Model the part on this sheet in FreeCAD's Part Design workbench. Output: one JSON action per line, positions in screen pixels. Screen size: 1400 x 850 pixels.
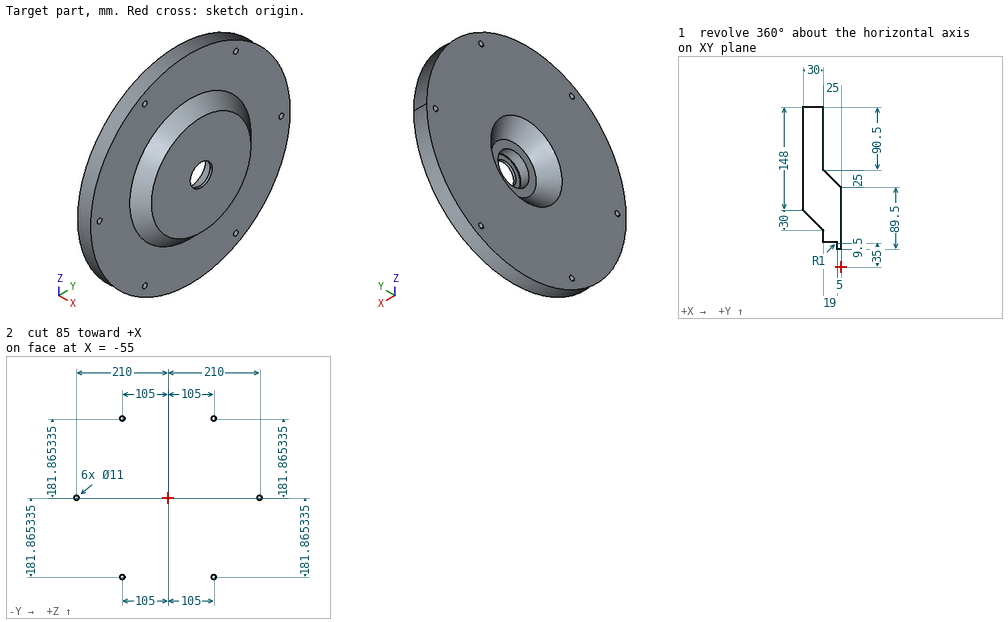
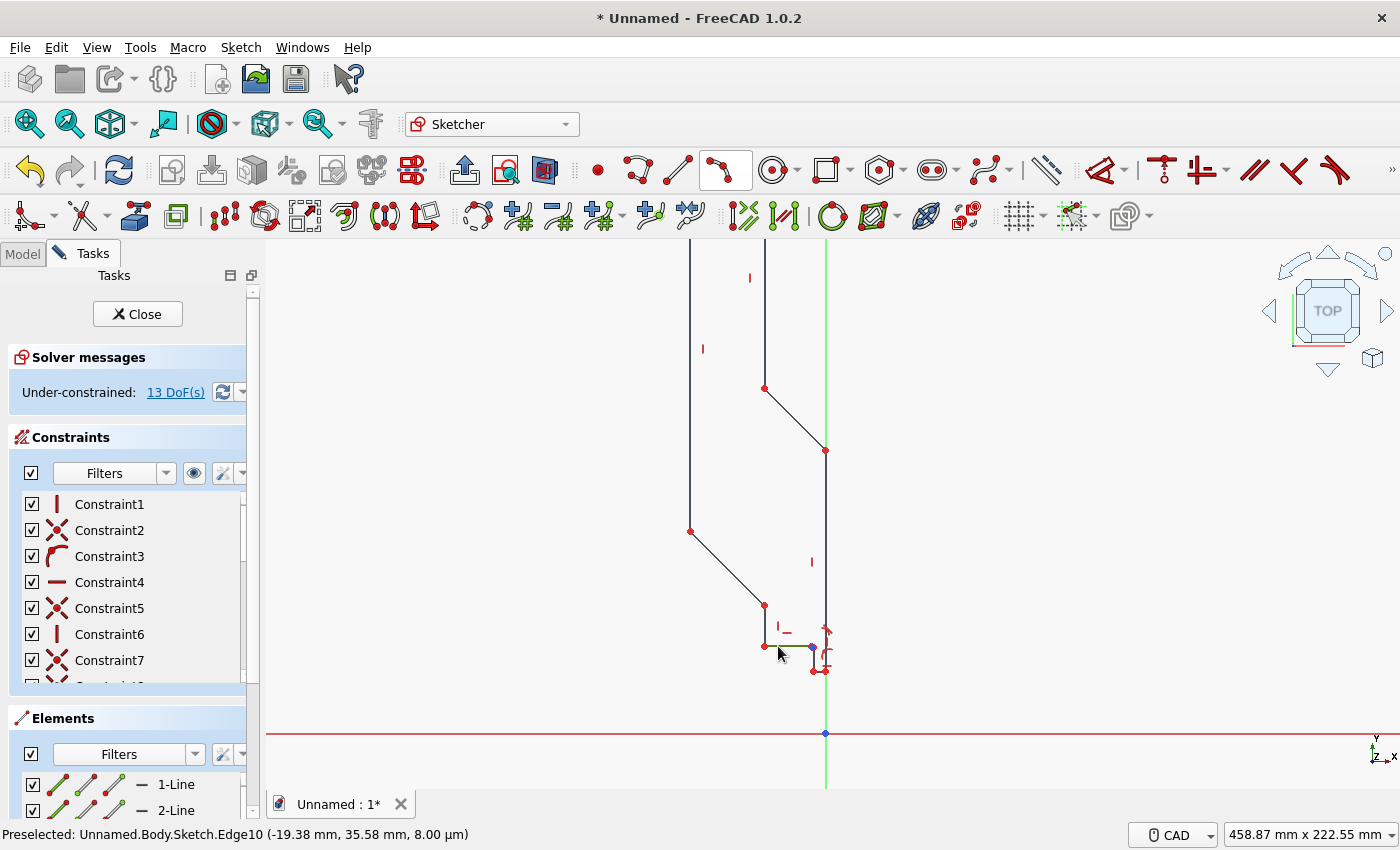
{"action": "scroll", "coordinate": [813, 646], "scroll_direction": "up", "scroll_amount": 11}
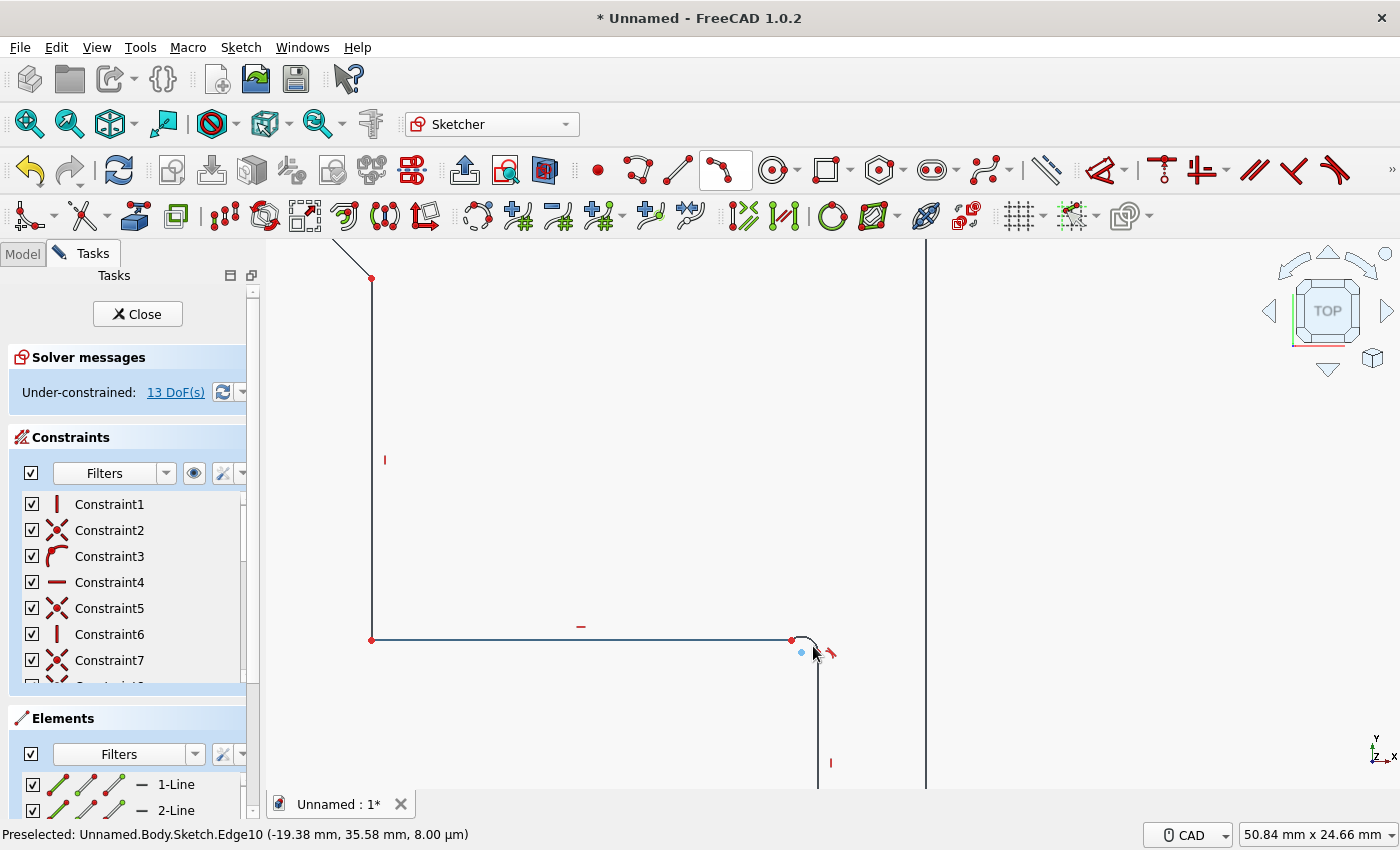
{"action": "left_click", "coordinate": [808, 638]}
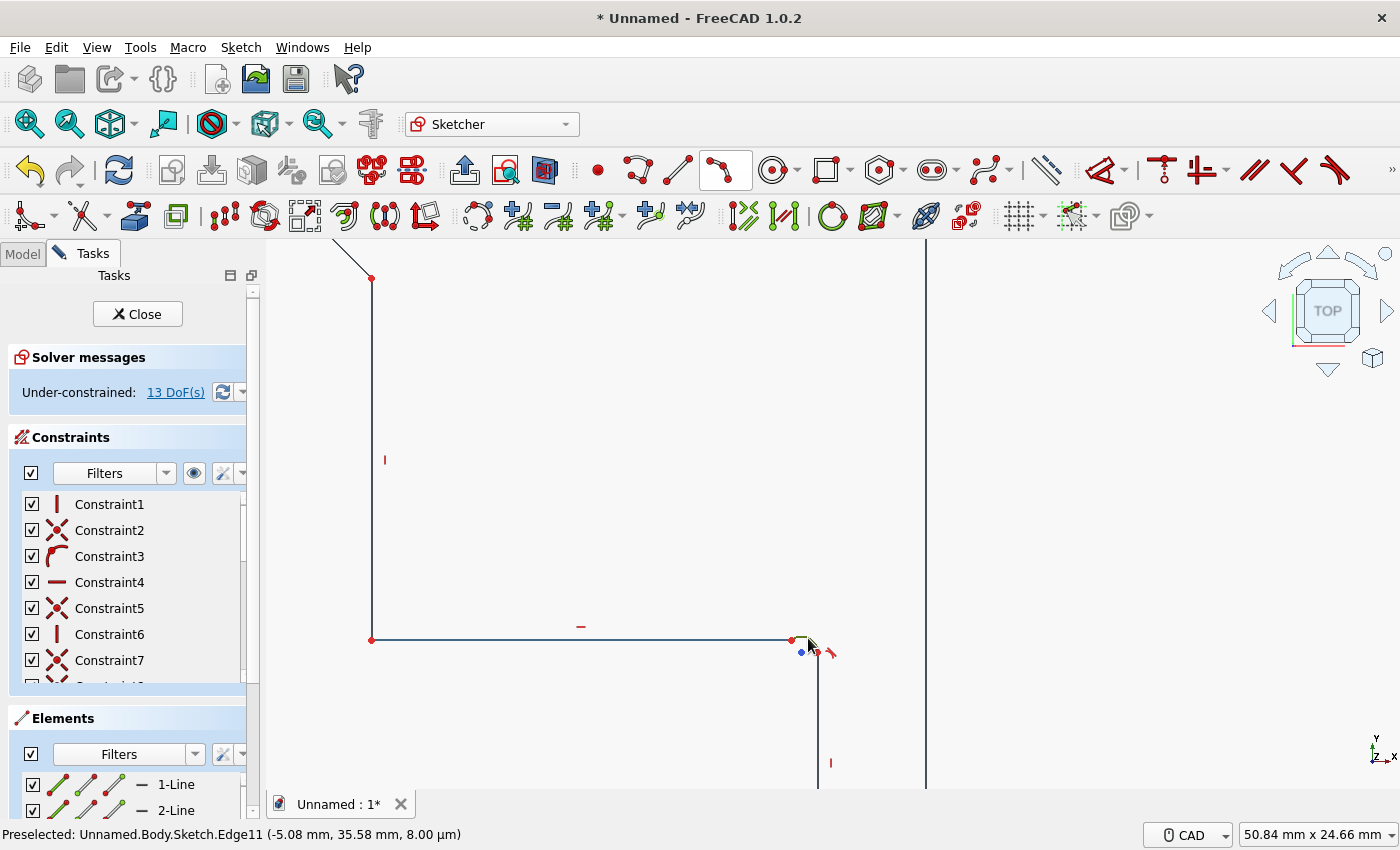
{"action": "left_click", "coordinate": [1336, 170]}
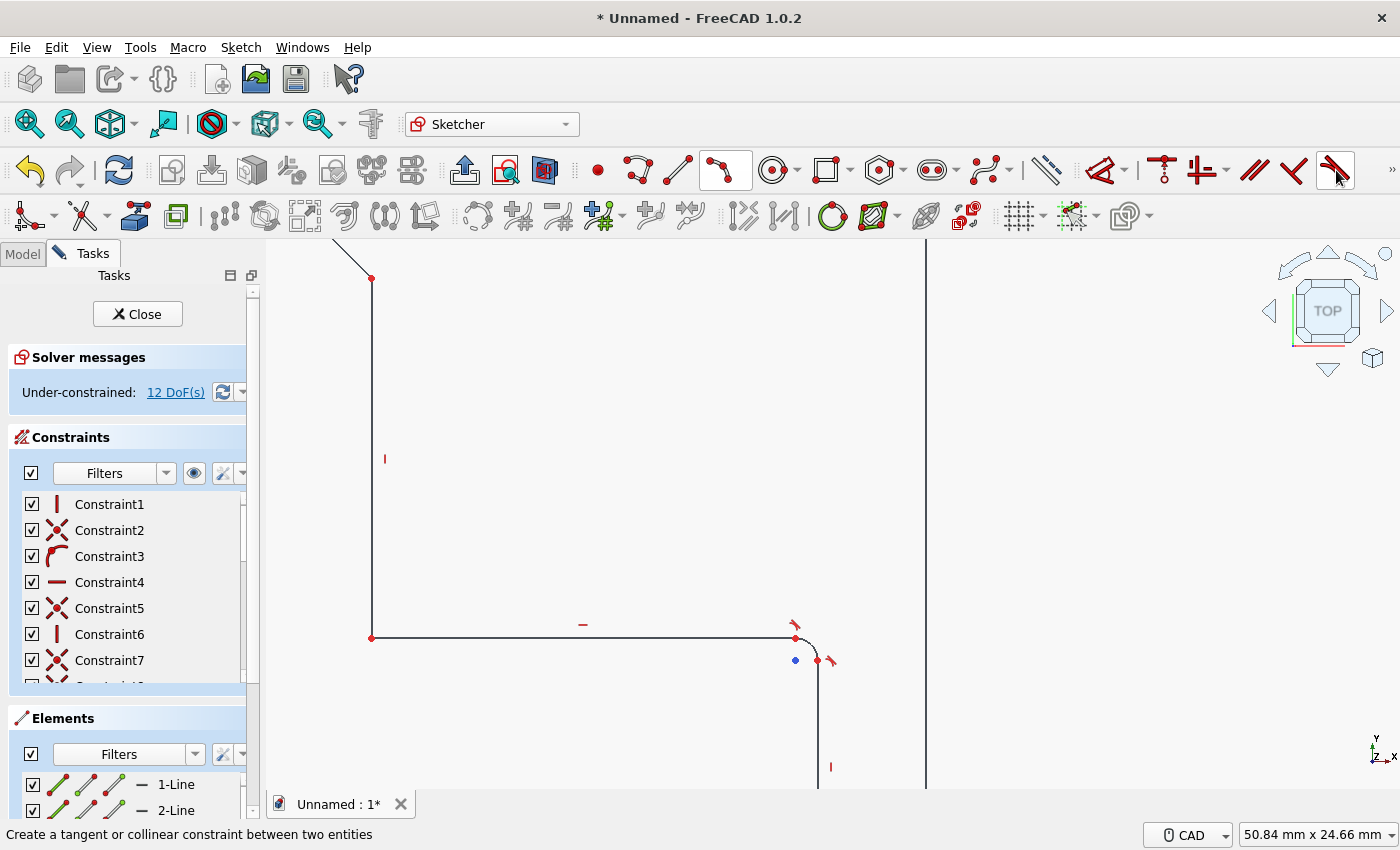
{"action": "left_click", "coordinate": [1100, 170]}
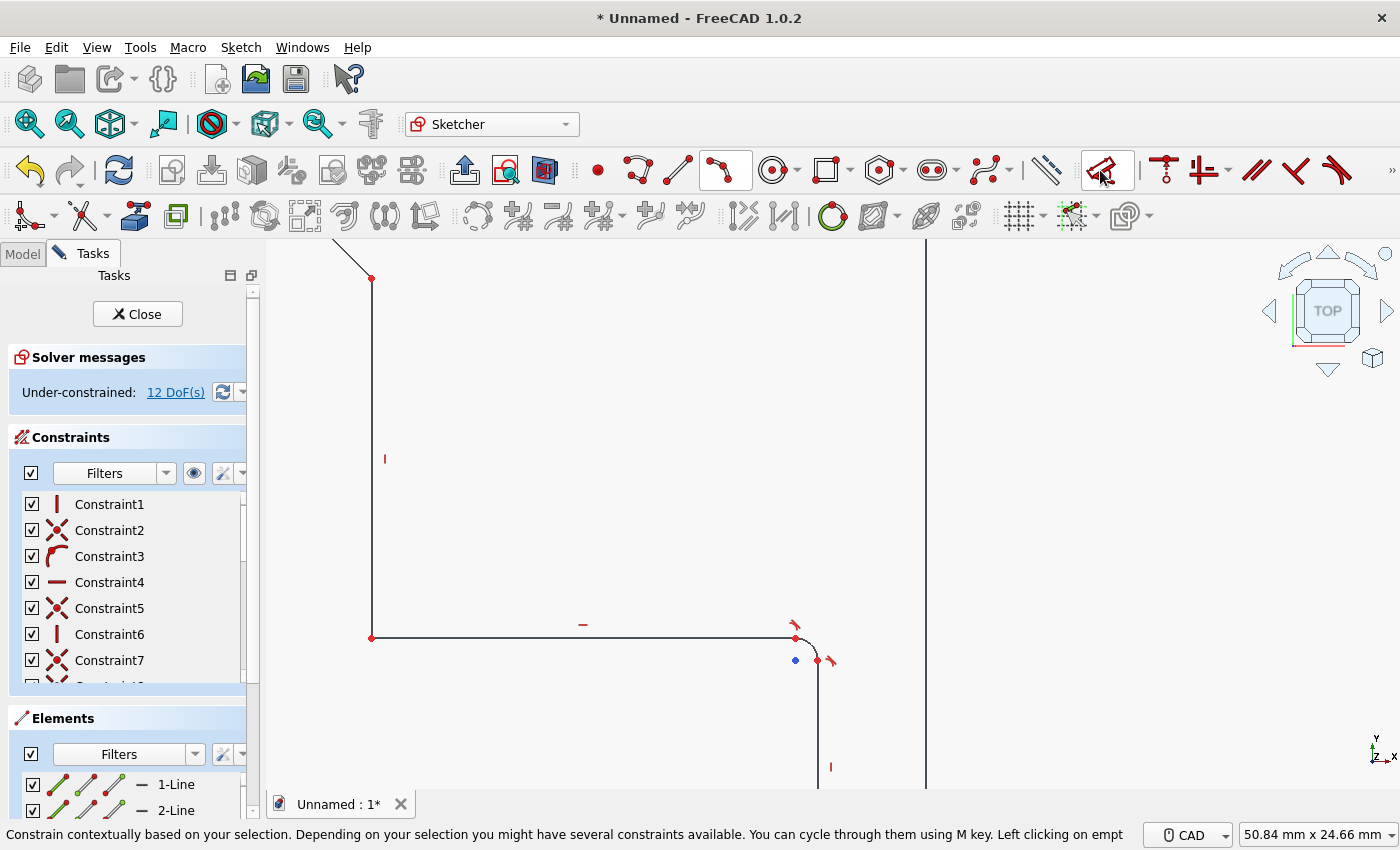
{"action": "scroll", "coordinate": [815, 651], "scroll_direction": "up", "scroll_amount": 3}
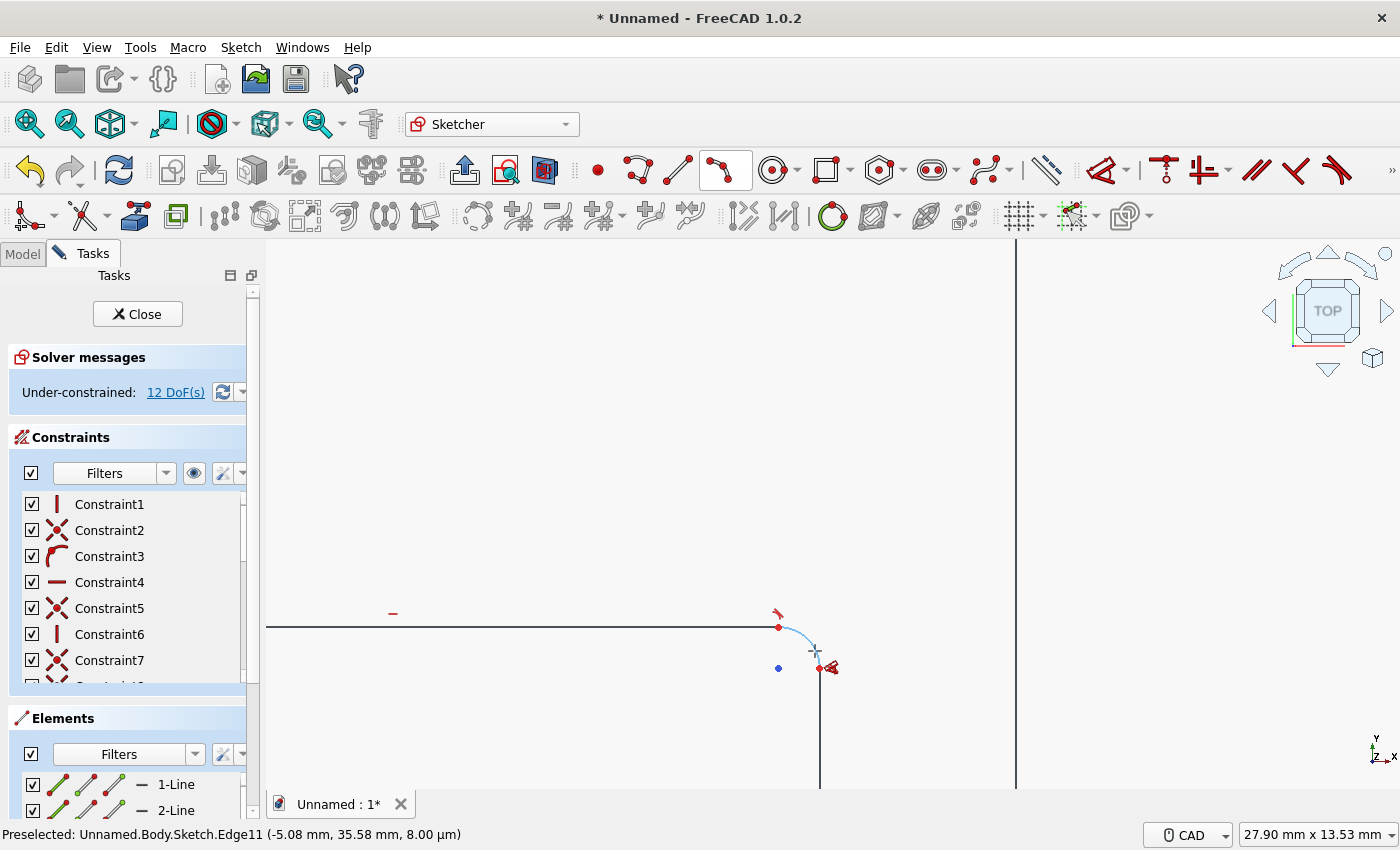
{"action": "left_click", "coordinate": [815, 650]}
{"action": "left_click", "coordinate": [844, 636]}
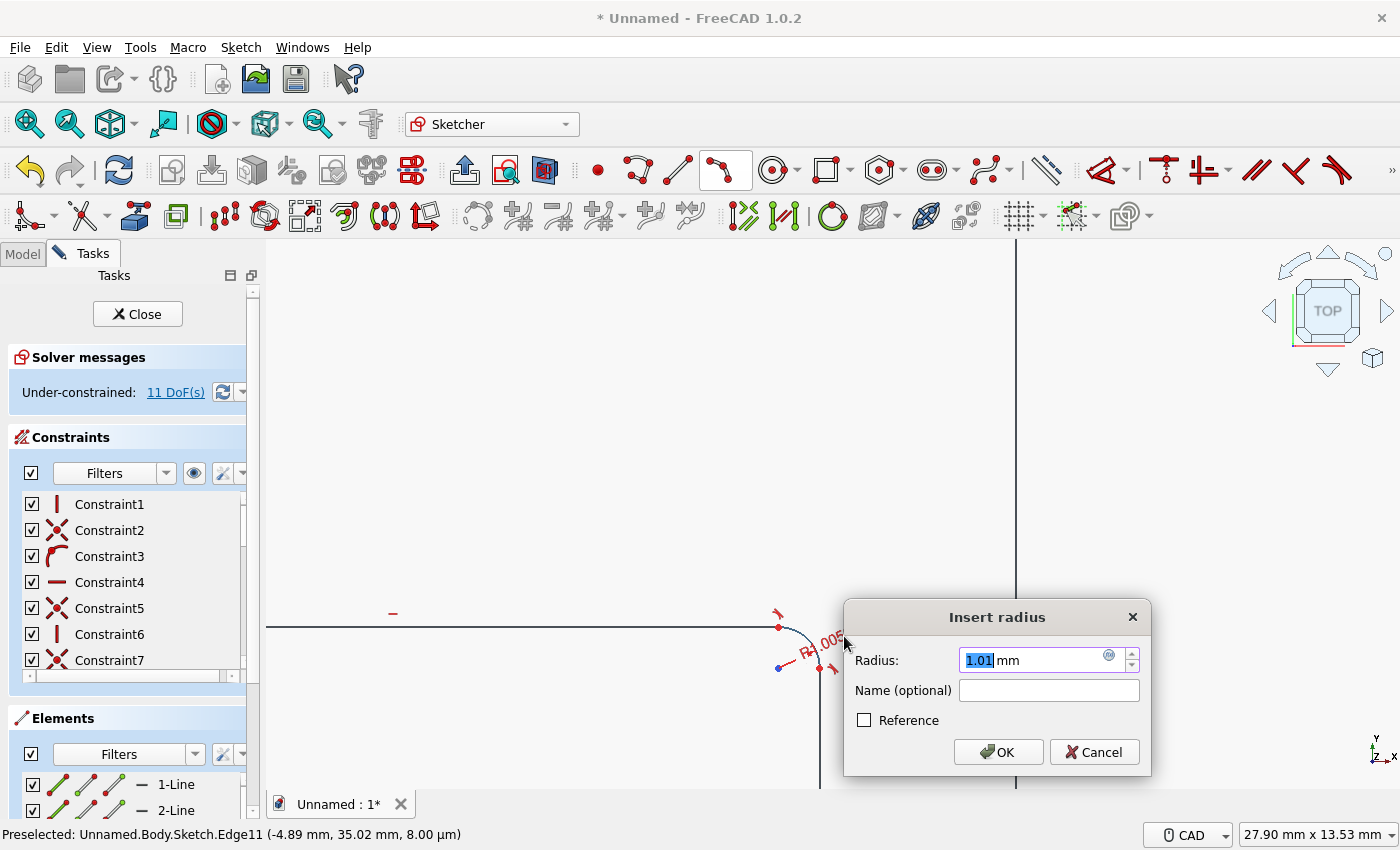
{"action": "type", "text": "1"}
{"action": "key", "text": "Return"}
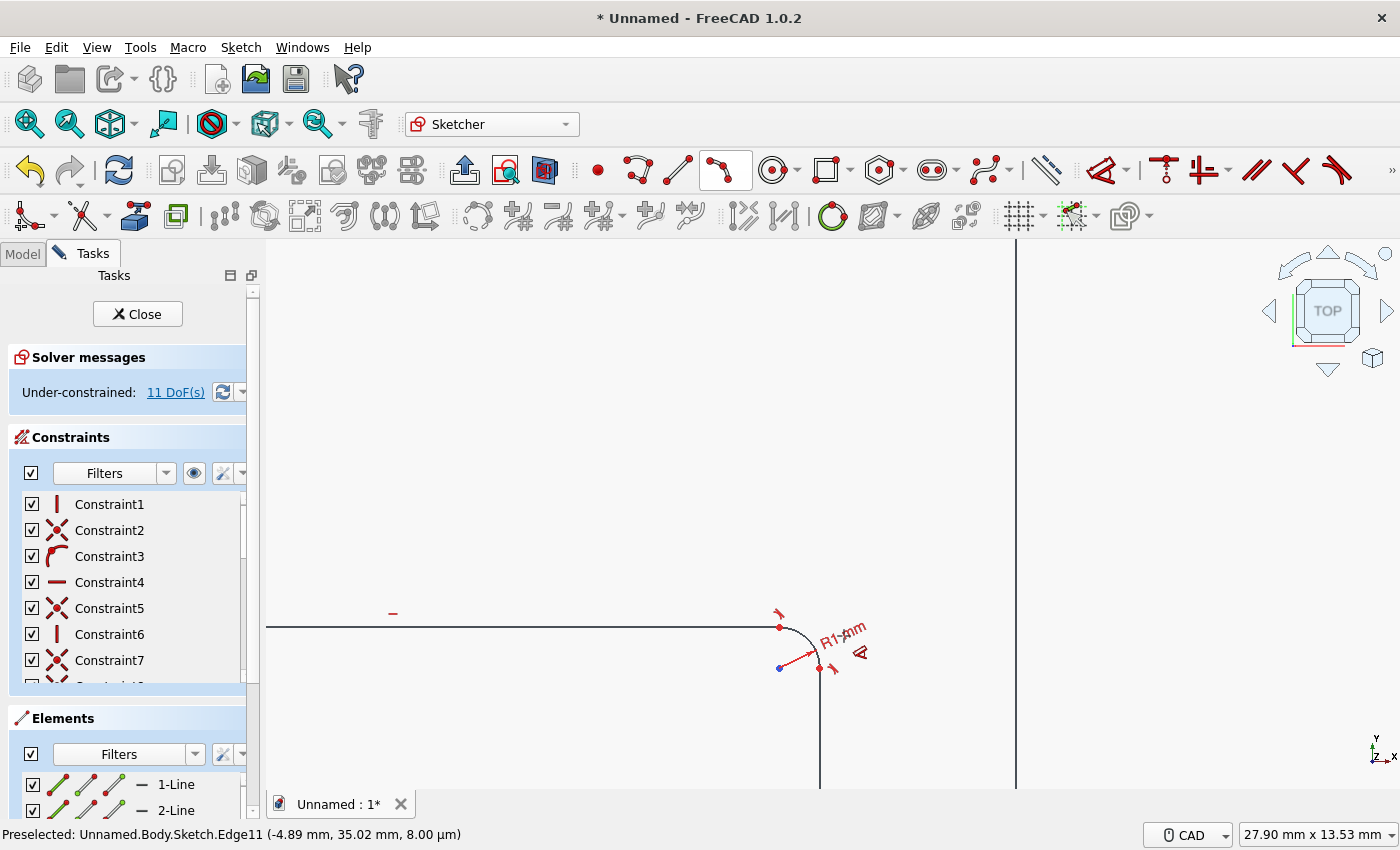
{"action": "scroll", "coordinate": [801, 647], "scroll_direction": "down", "scroll_amount": 16}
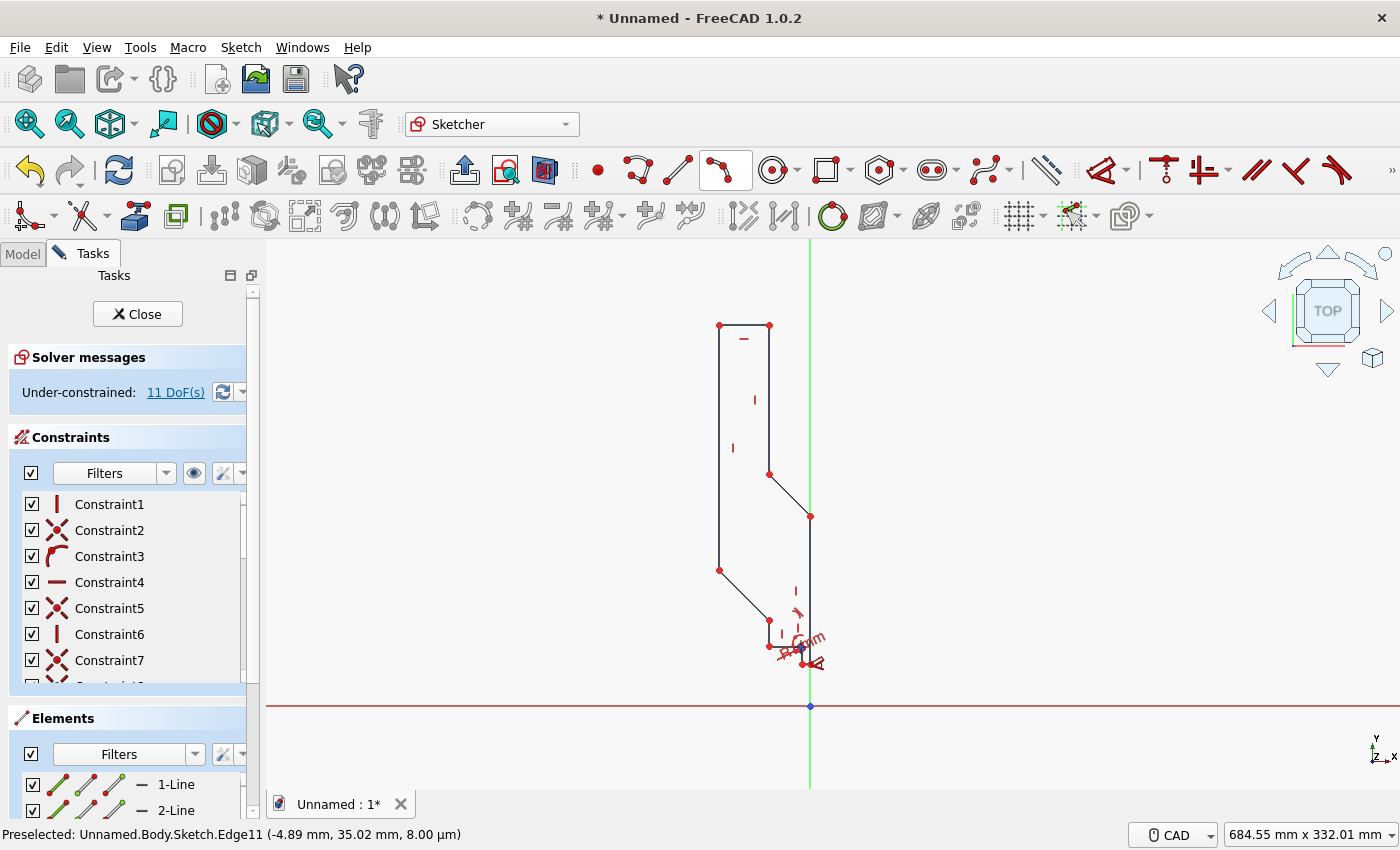
{"action": "scroll", "coordinate": [805, 664], "scroll_direction": "up", "scroll_amount": 9}